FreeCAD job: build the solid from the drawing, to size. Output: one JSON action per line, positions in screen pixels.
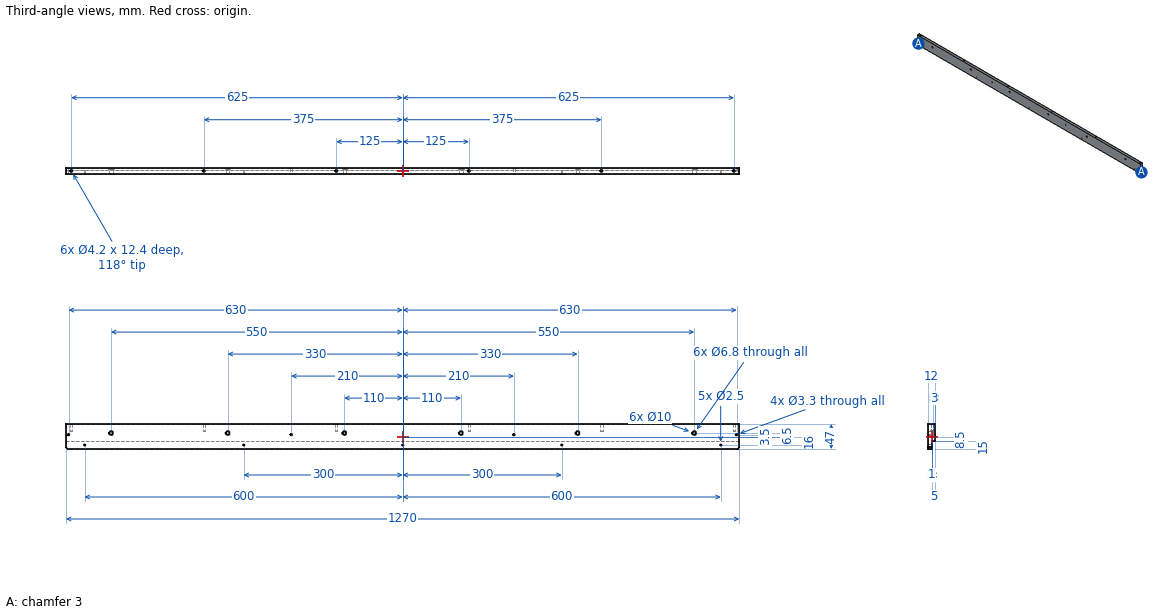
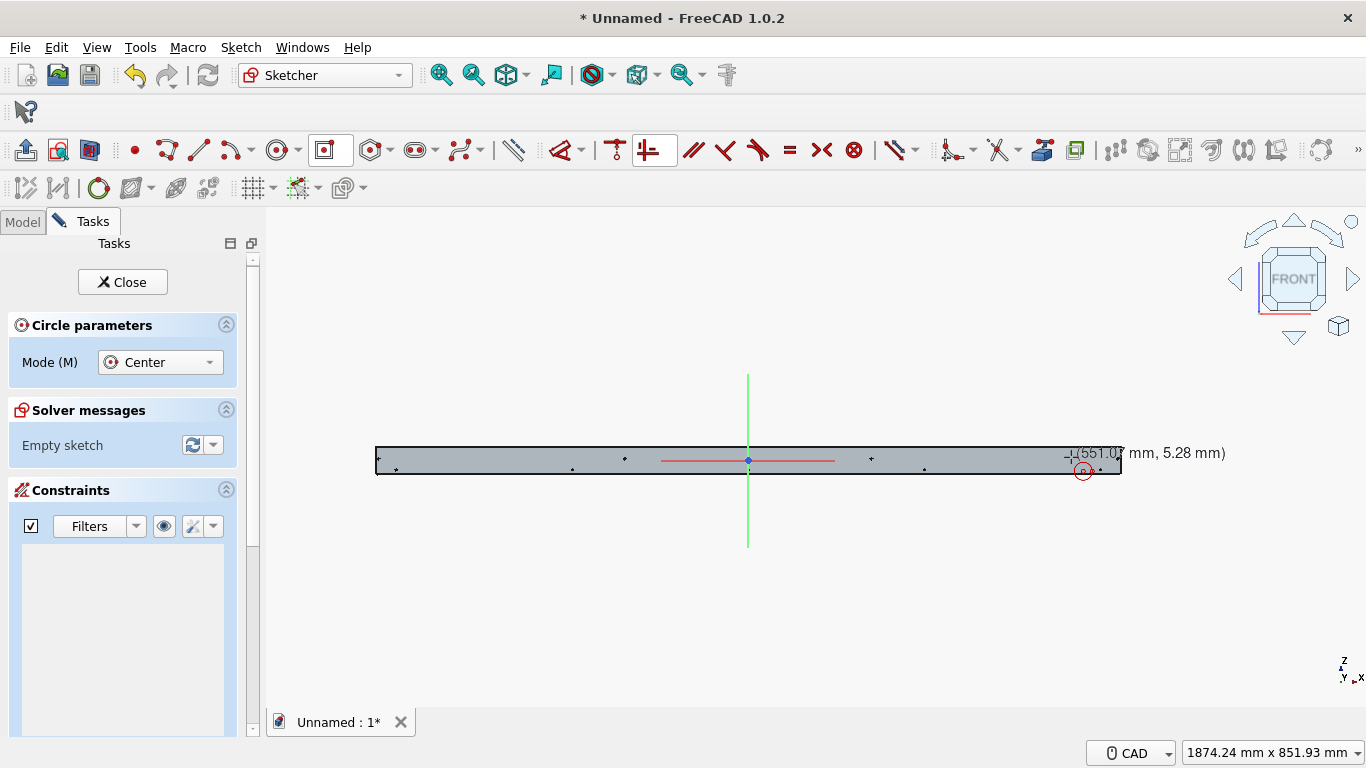
{"action": "scroll", "coordinate": [1071, 457], "scroll_direction": "up", "scroll_amount": 8}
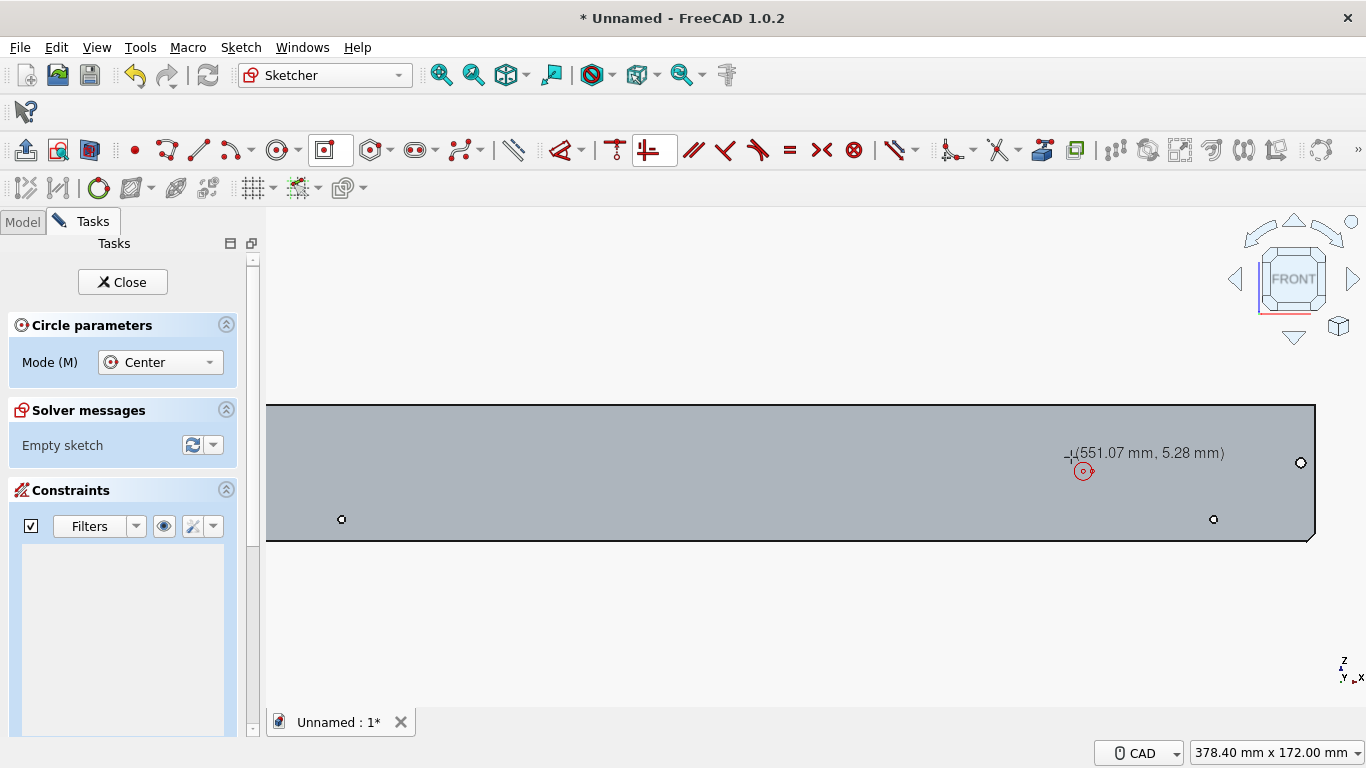
{"action": "left_click", "coordinate": [1068, 454]}
{"action": "mouse_move", "coordinate": [1075, 447]}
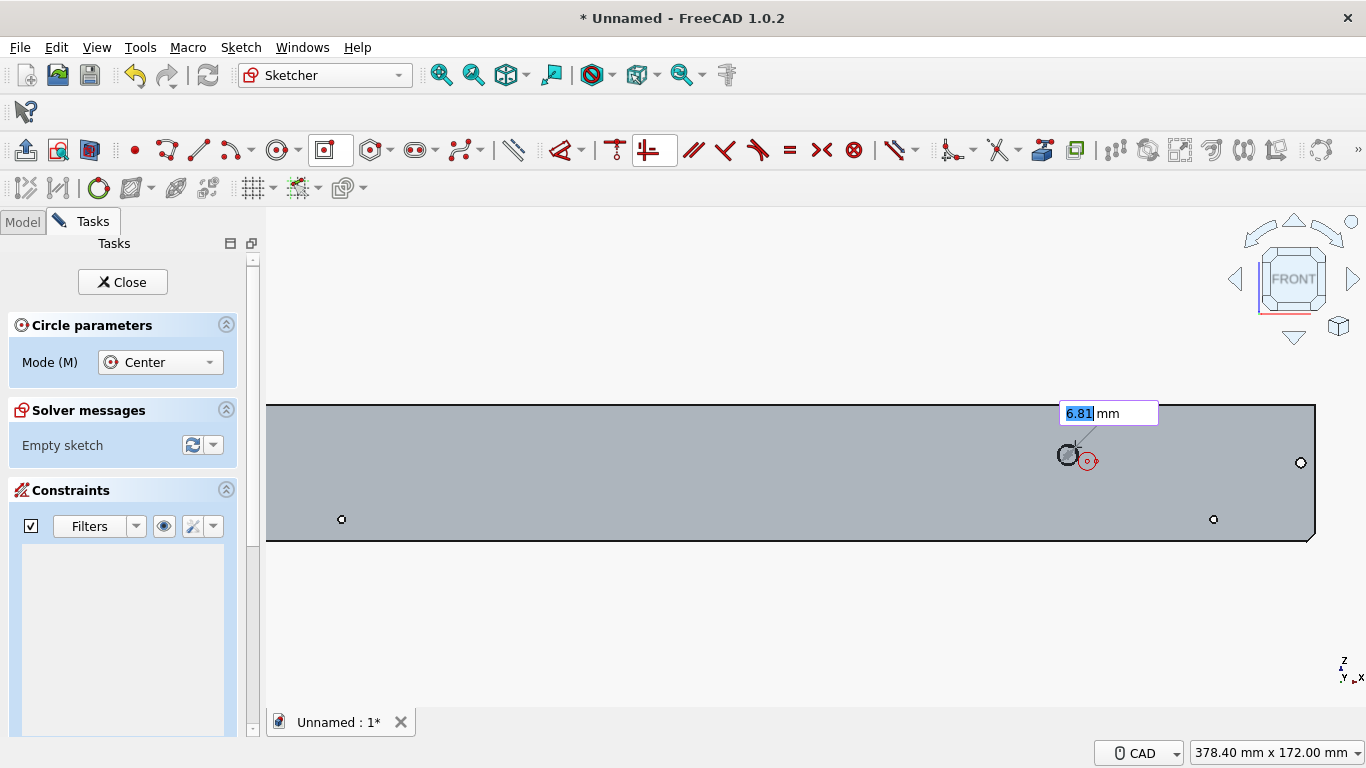
{"action": "type", "text": "6.8"}
{"action": "key", "text": "Return"}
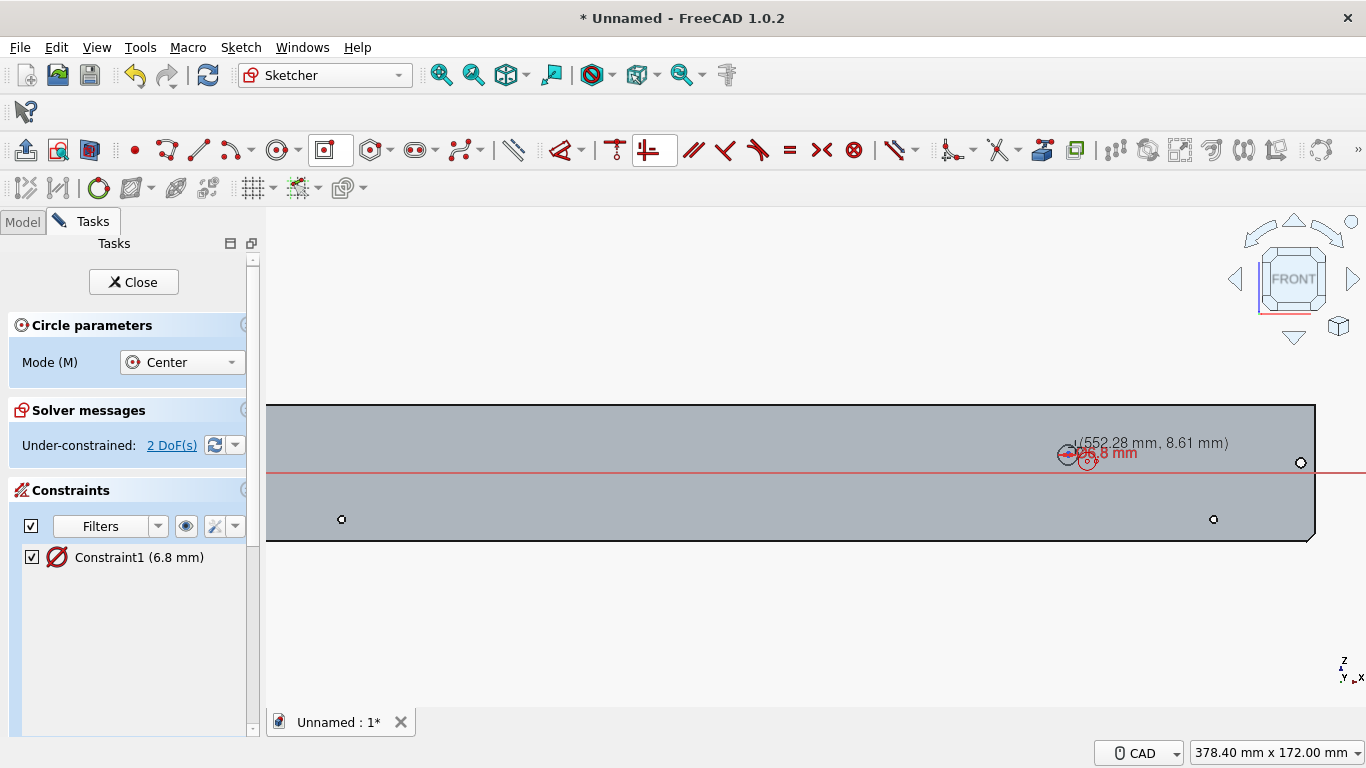
{"action": "scroll", "coordinate": [429, 454], "scroll_direction": "up", "scroll_amount": 5}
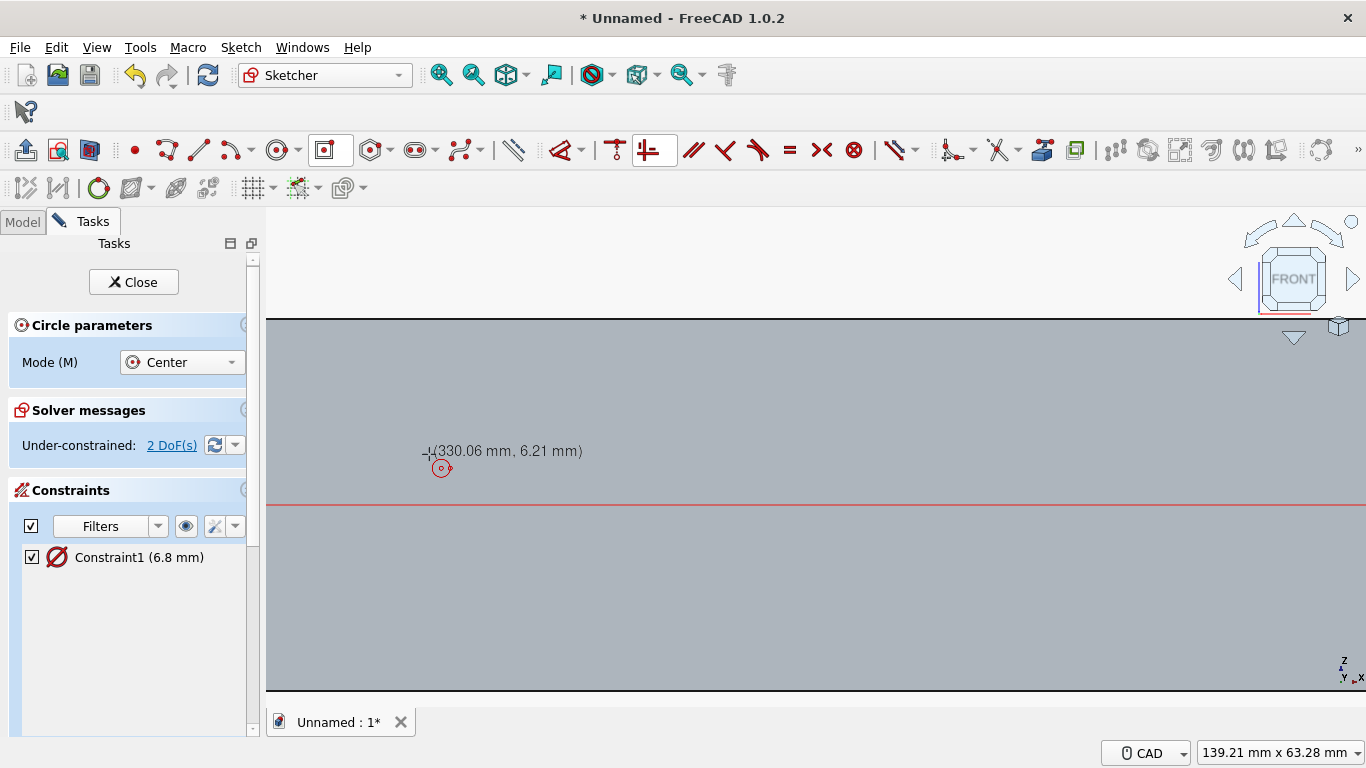
{"action": "scroll", "coordinate": [982, 456], "scroll_direction": "down", "scroll_amount": 13}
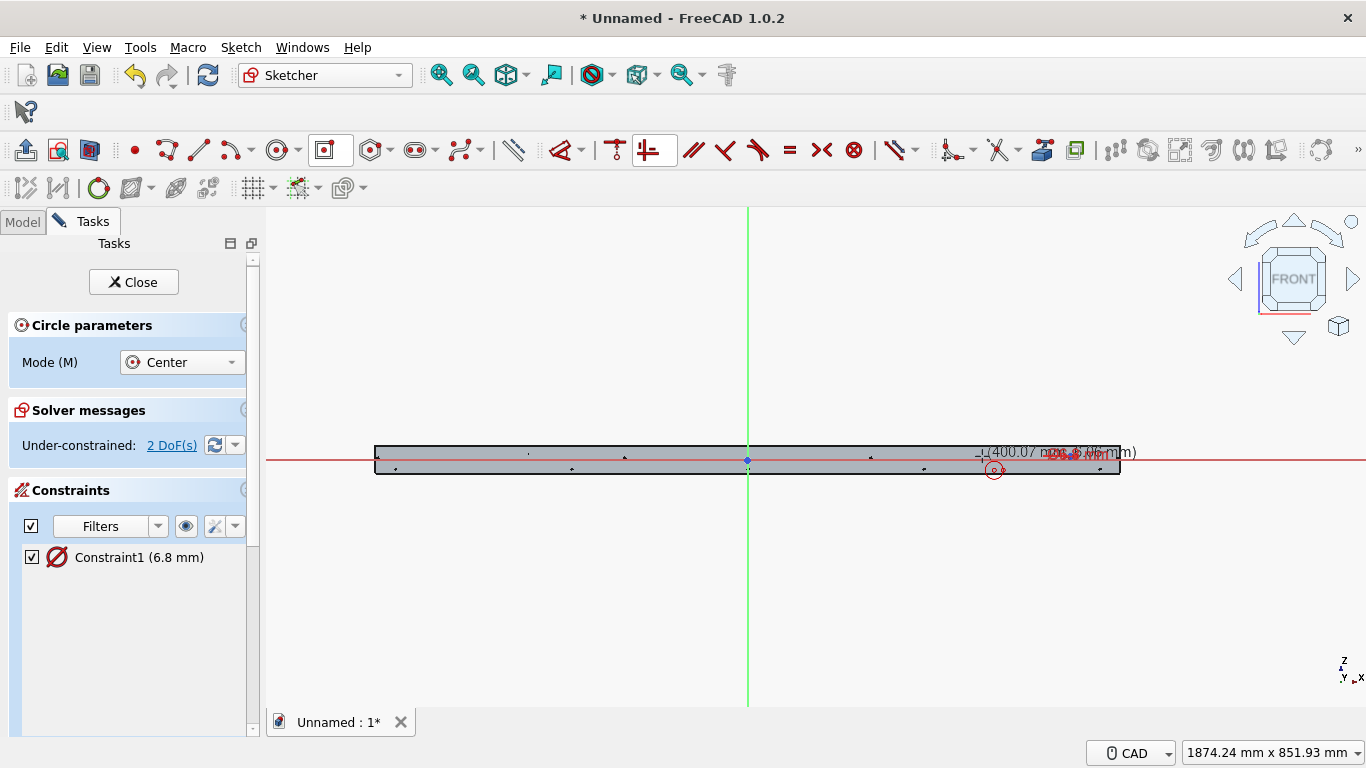
{"action": "scroll", "coordinate": [941, 456], "scroll_direction": "up", "scroll_amount": 8}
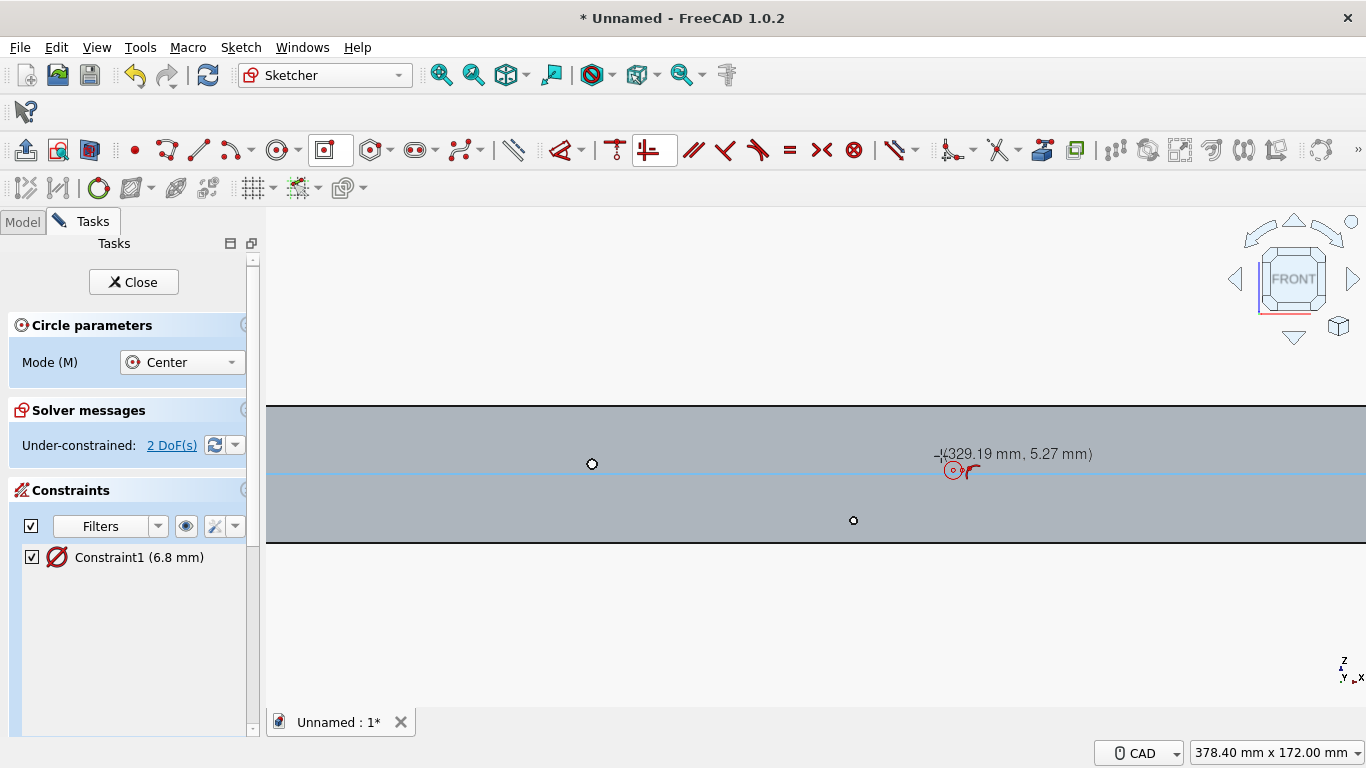
{"action": "left_click", "coordinate": [941, 455]}
{"action": "mouse_move", "coordinate": [948, 448]}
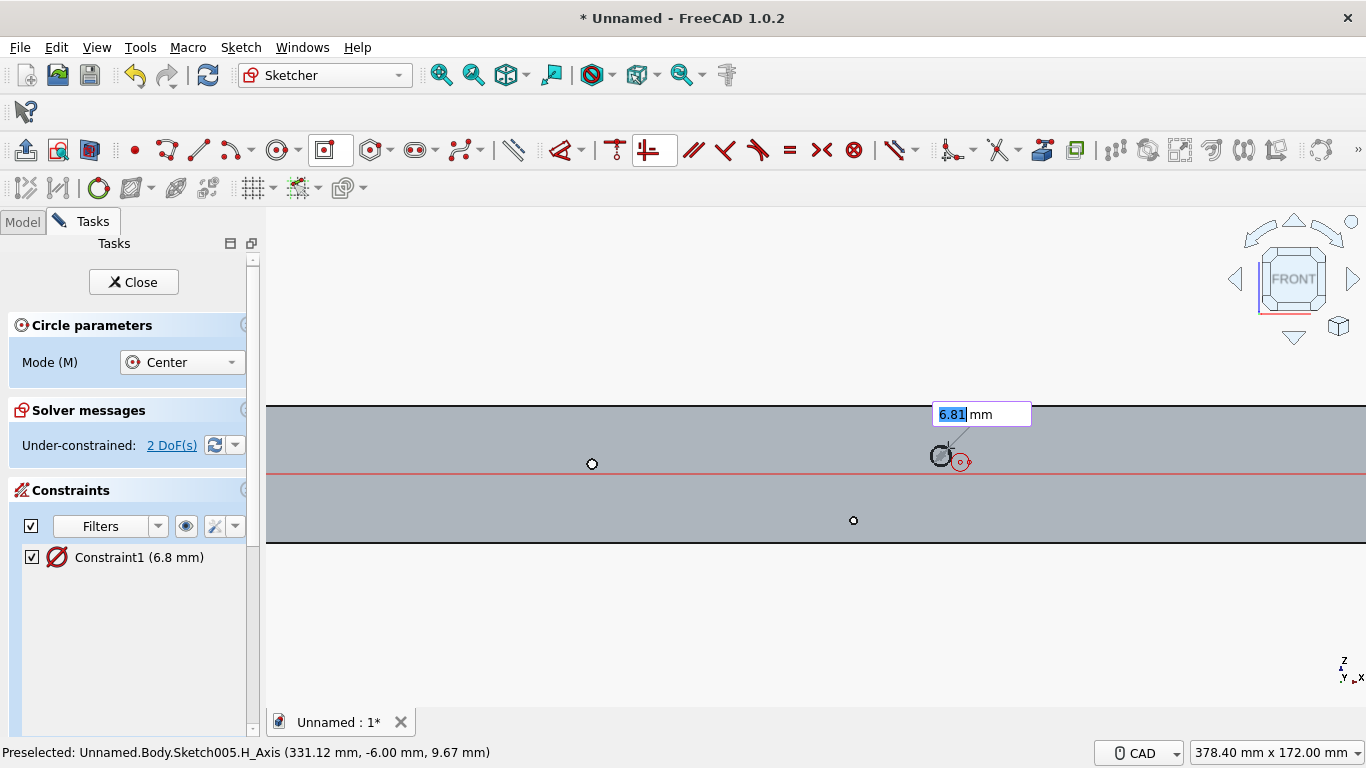
{"action": "type", "text": "6.8"}
{"action": "key", "text": "Return"}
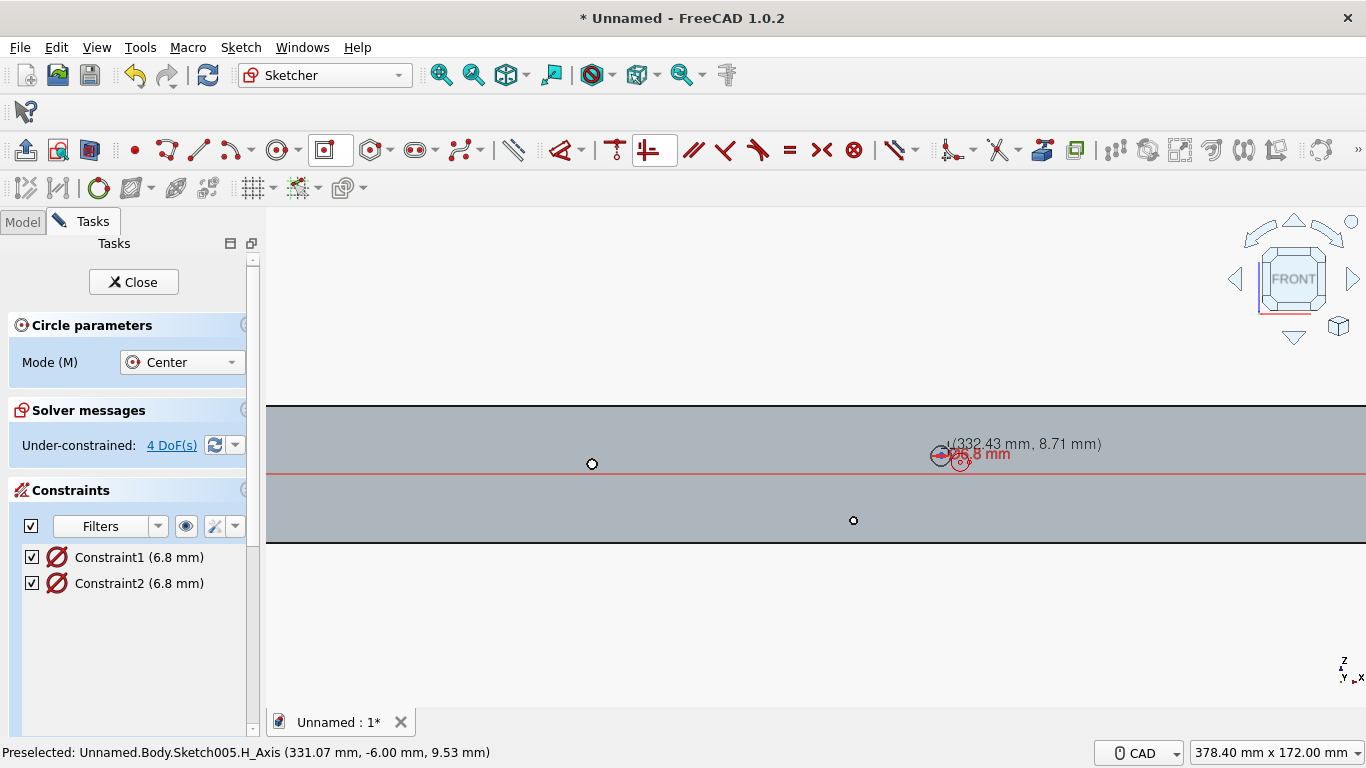
{"action": "scroll", "coordinate": [301, 455], "scroll_direction": "up", "scroll_amount": 5}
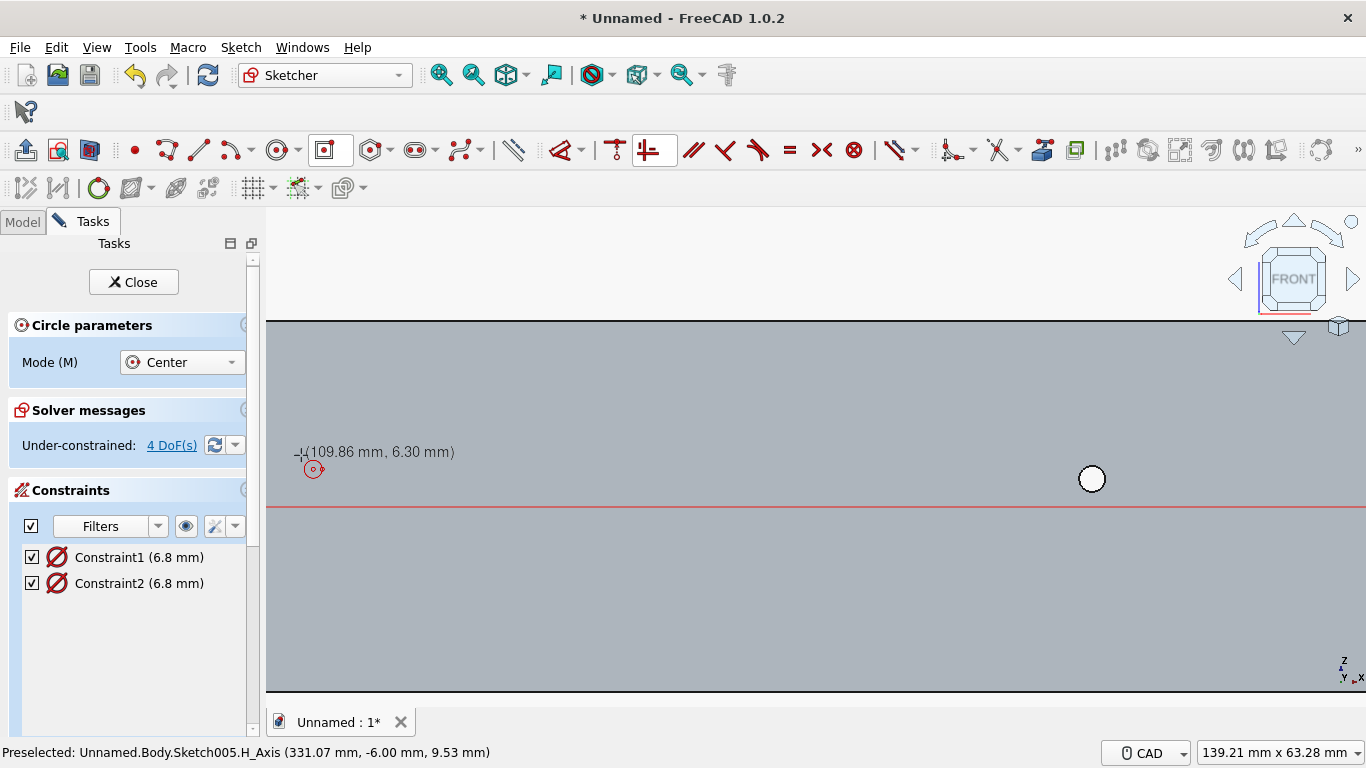
{"action": "scroll", "coordinate": [853, 456], "scroll_direction": "down", "scroll_amount": 13}